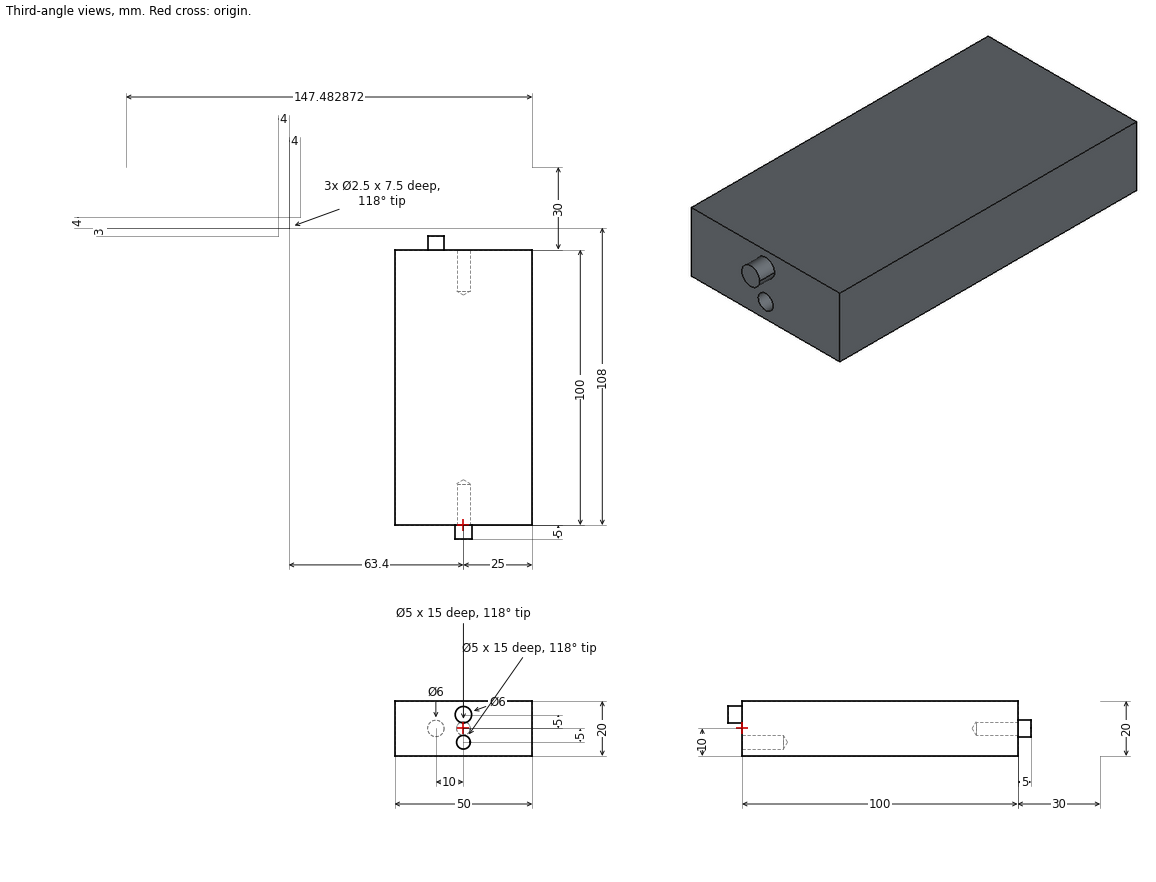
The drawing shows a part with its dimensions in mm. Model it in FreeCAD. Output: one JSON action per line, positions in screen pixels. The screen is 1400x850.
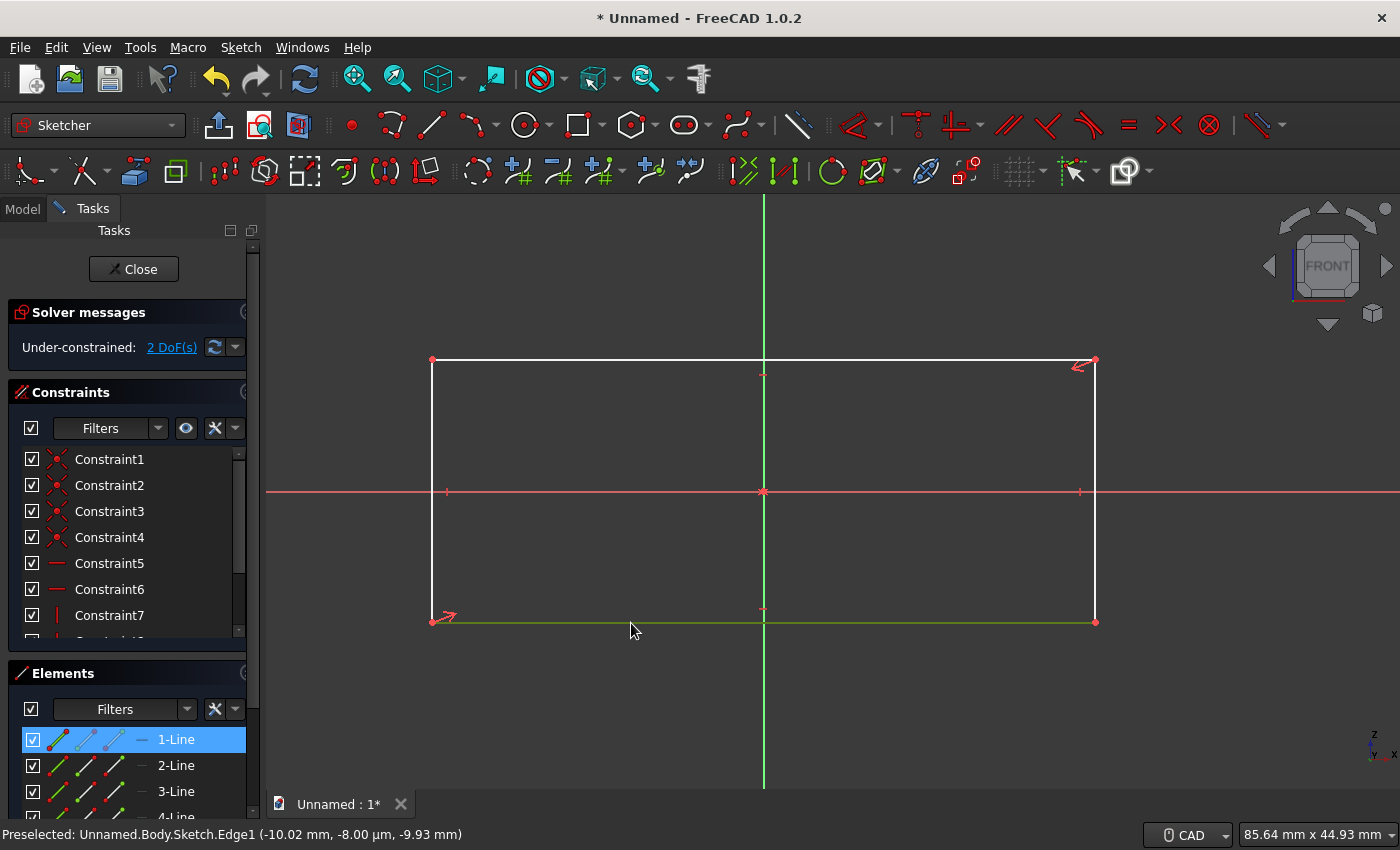
{"action": "key", "text": "l"}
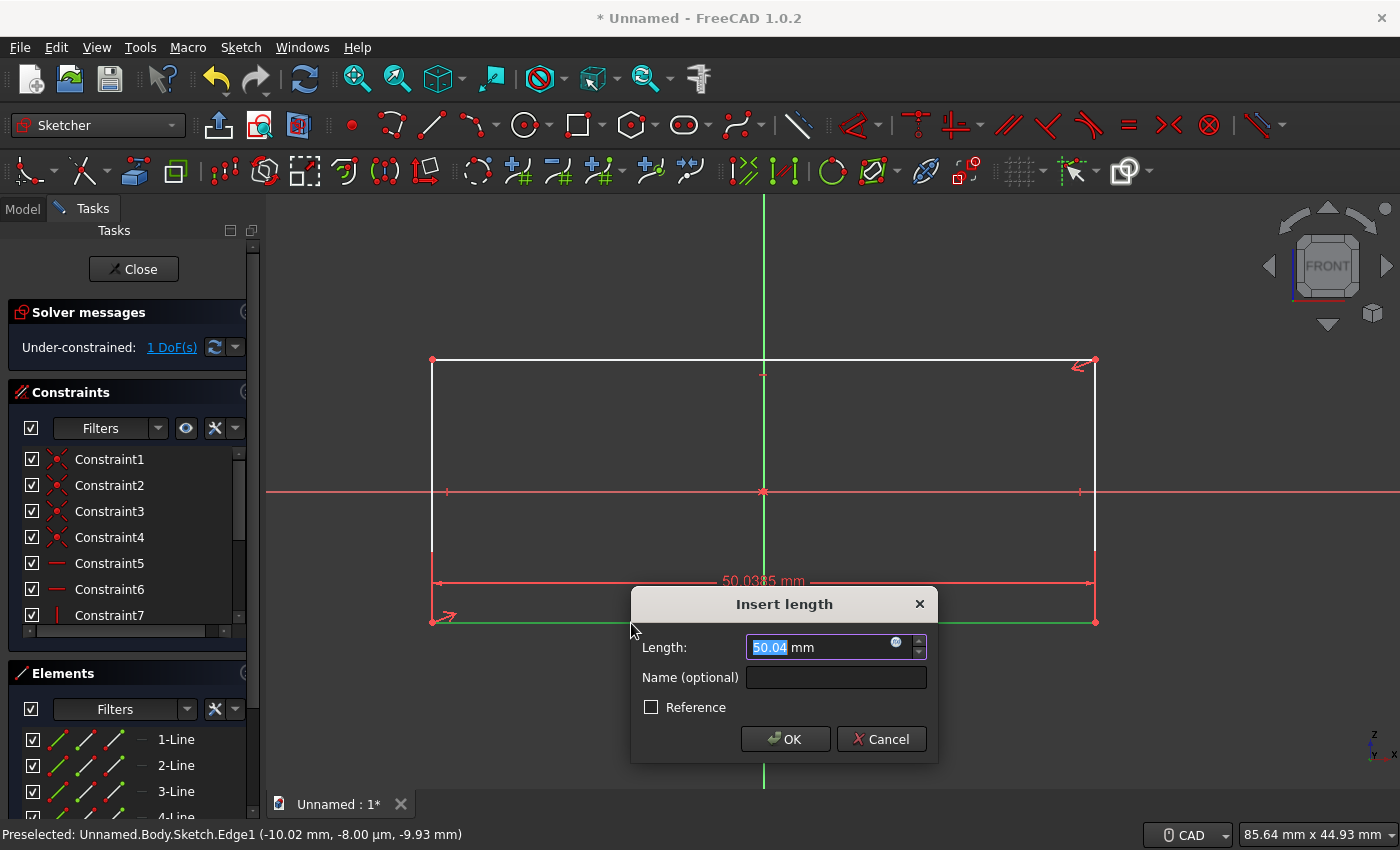
{"action": "type", "text": "50"}
{"action": "key", "text": "Return"}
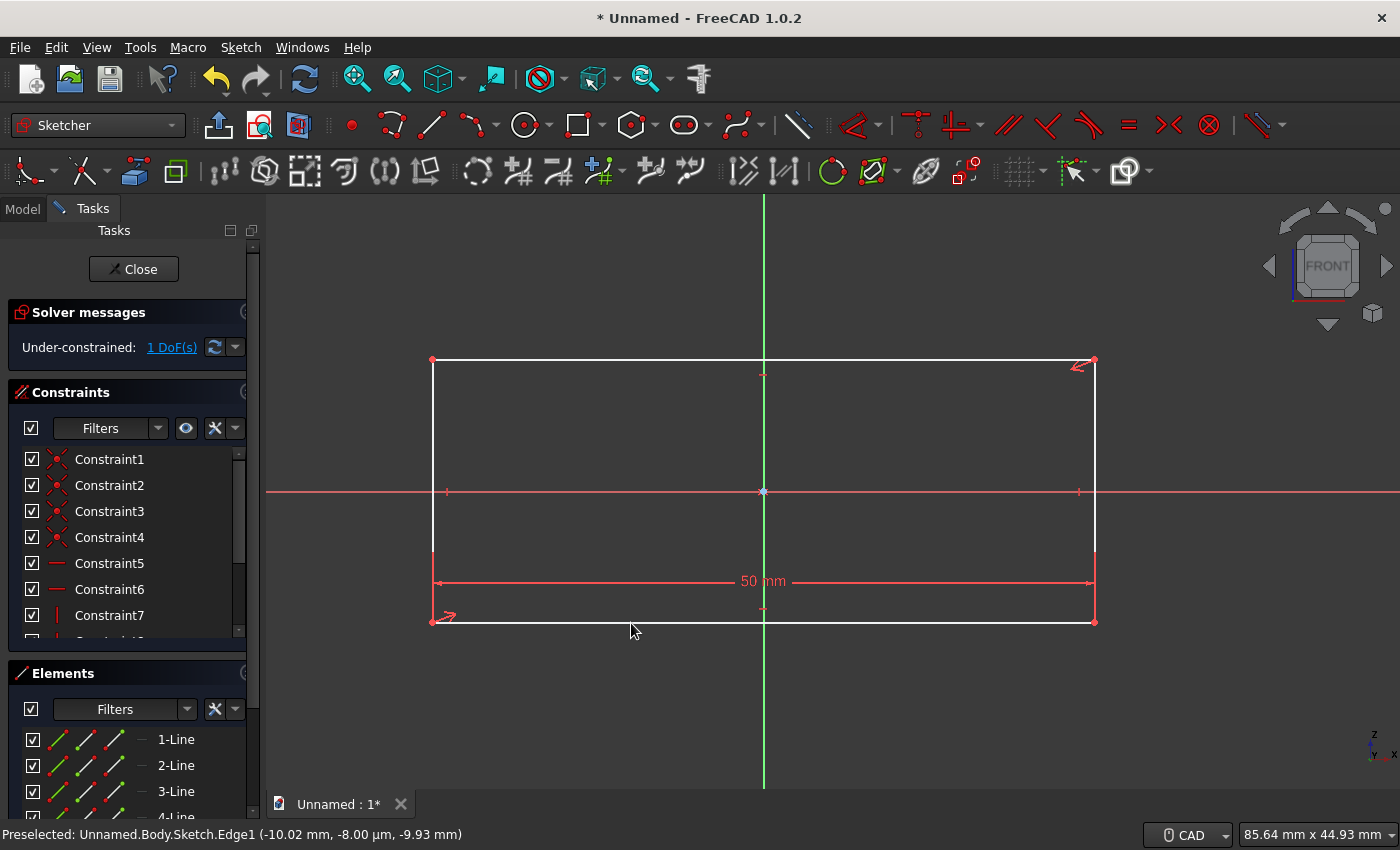
{"action": "left_click", "coordinate": [1095, 544]}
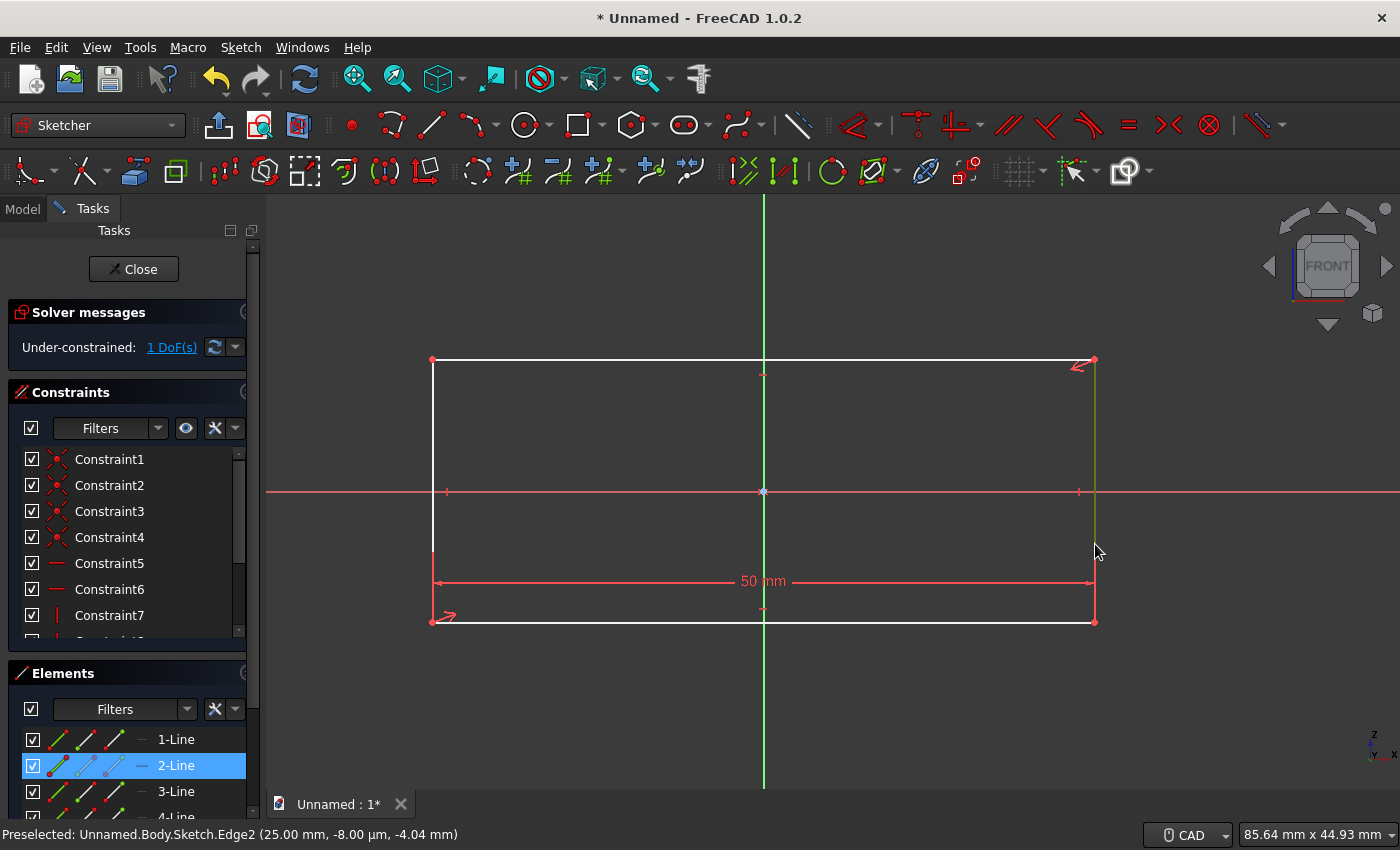
{"action": "left_click", "coordinate": [880, 126]}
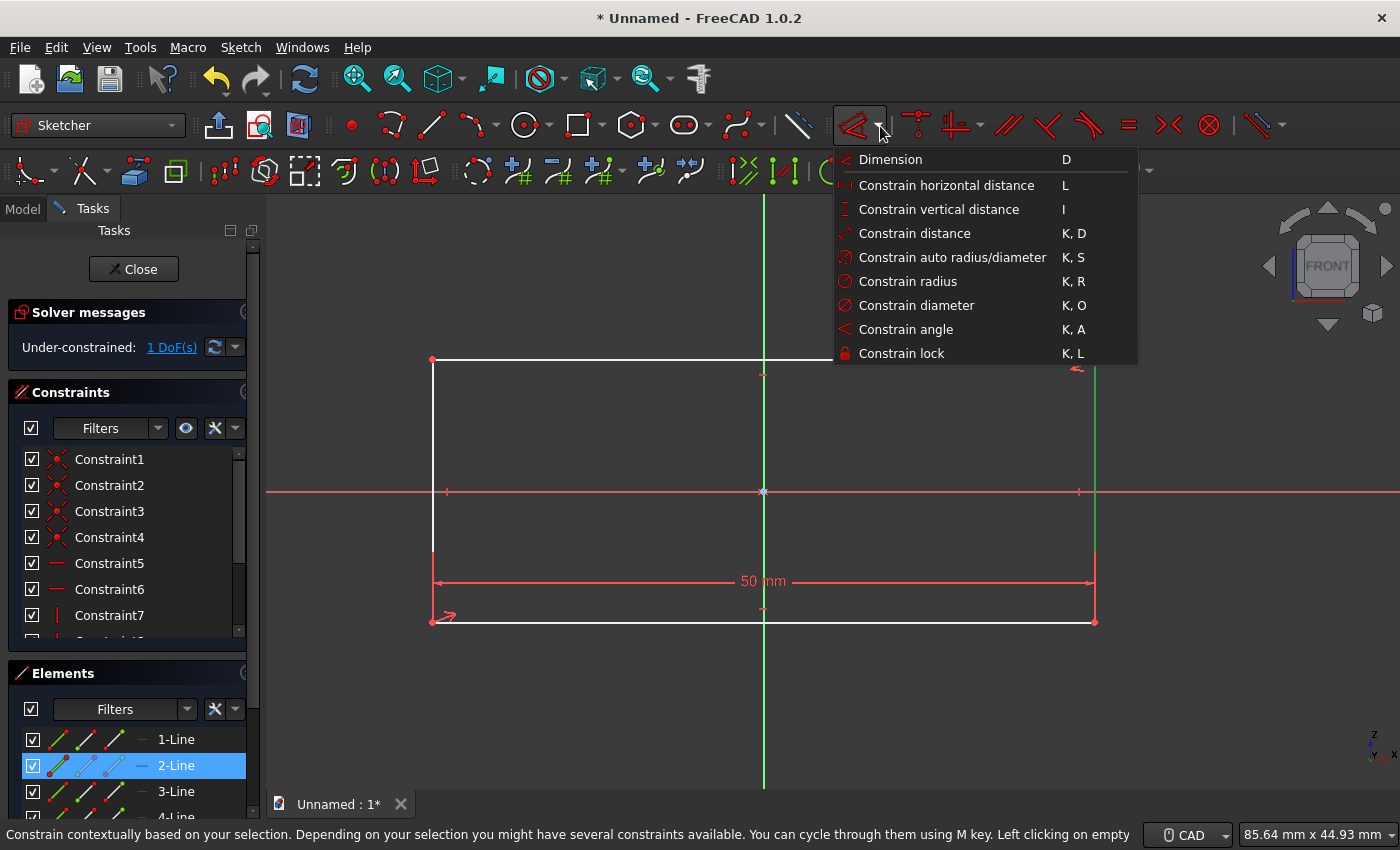
{"action": "left_click", "coordinate": [986, 209]}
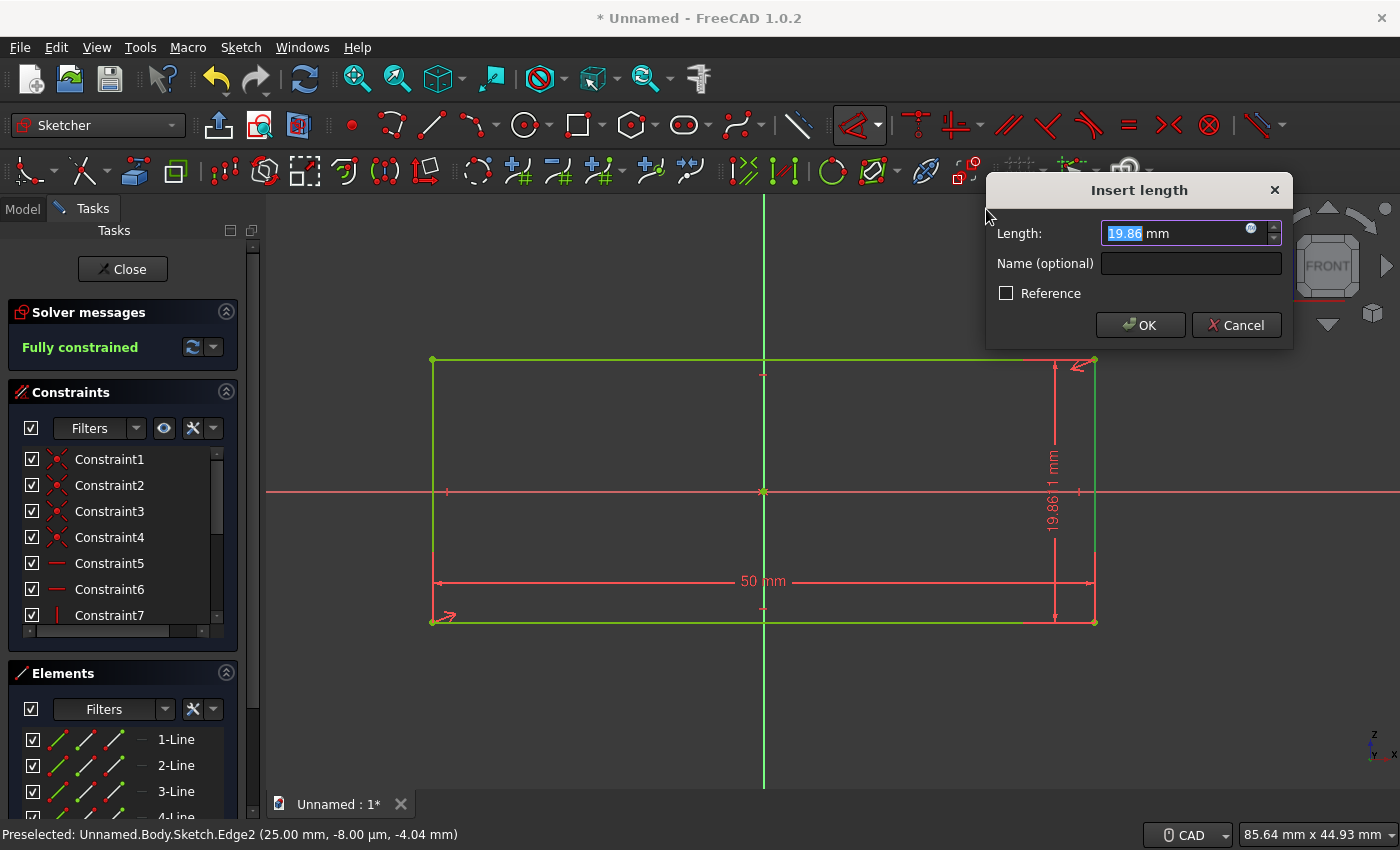
{"action": "type", "text": "20"}
{"action": "key", "text": "Return"}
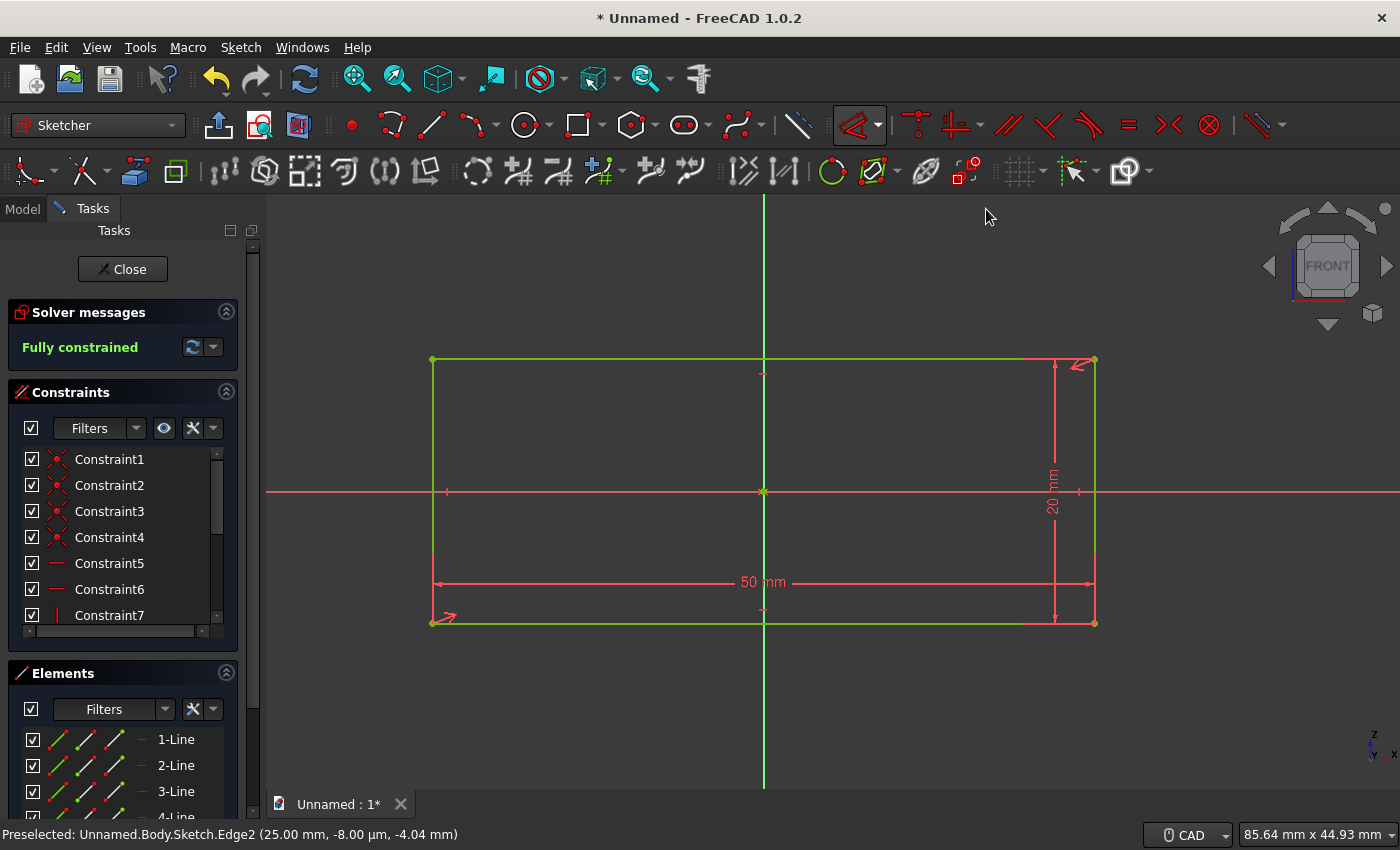
{"action": "left_click", "coordinate": [123, 269]}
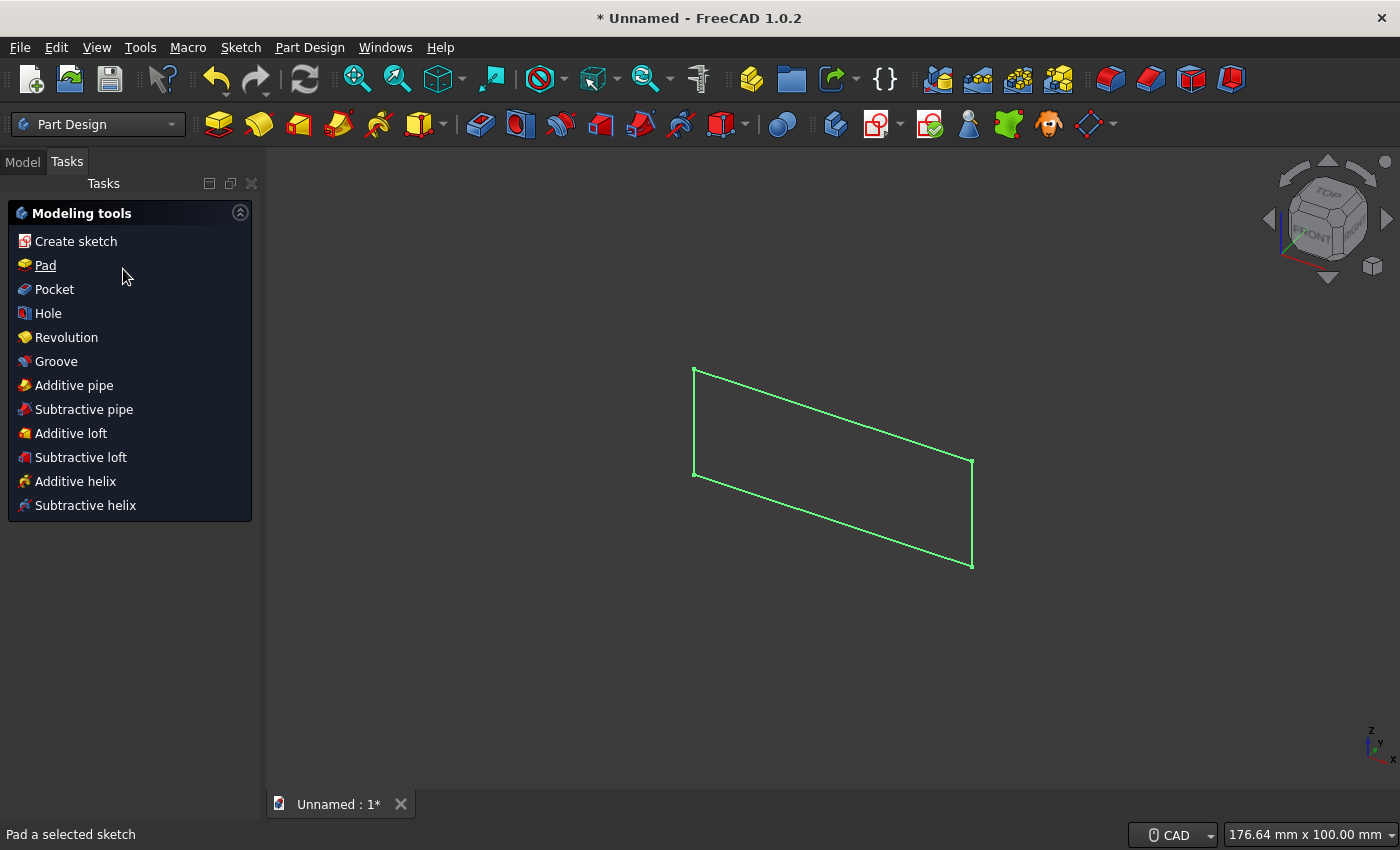
{"action": "left_click", "coordinate": [220, 124]}